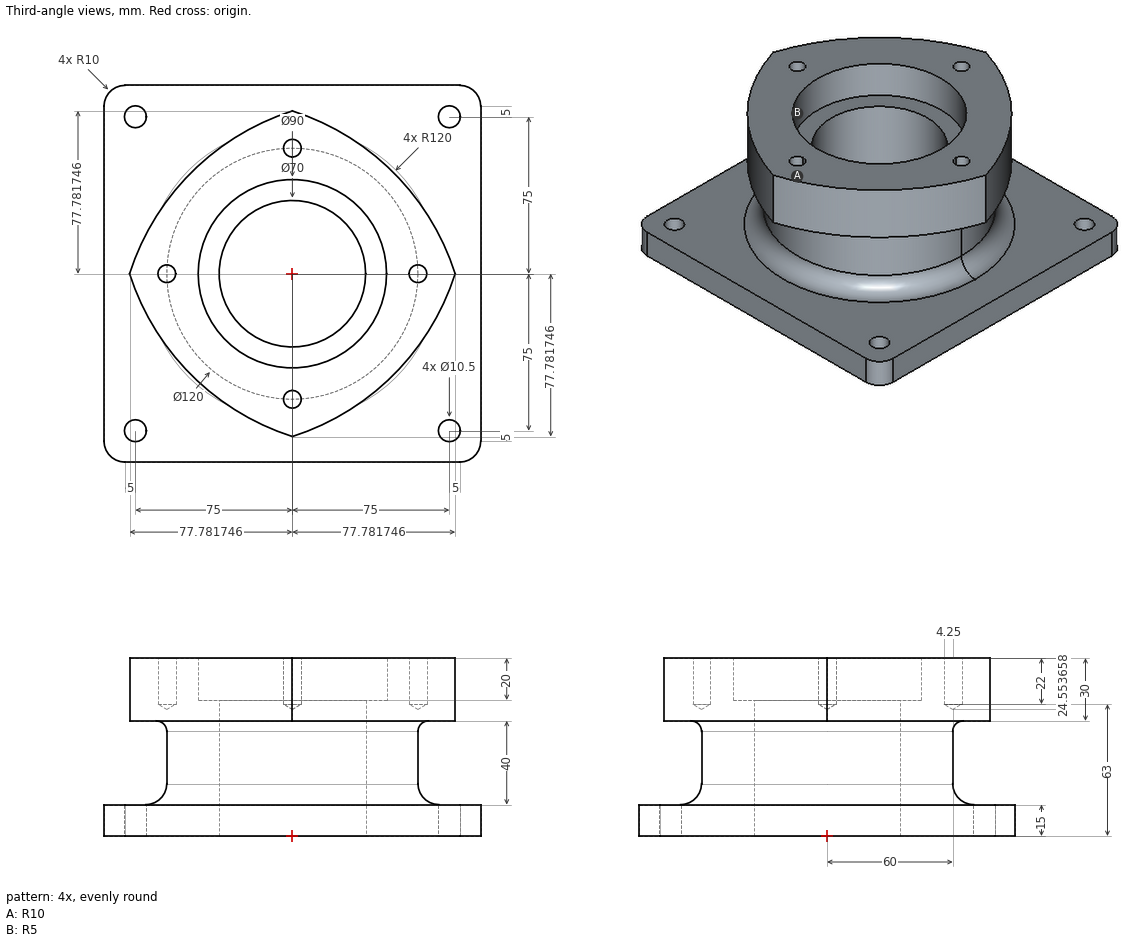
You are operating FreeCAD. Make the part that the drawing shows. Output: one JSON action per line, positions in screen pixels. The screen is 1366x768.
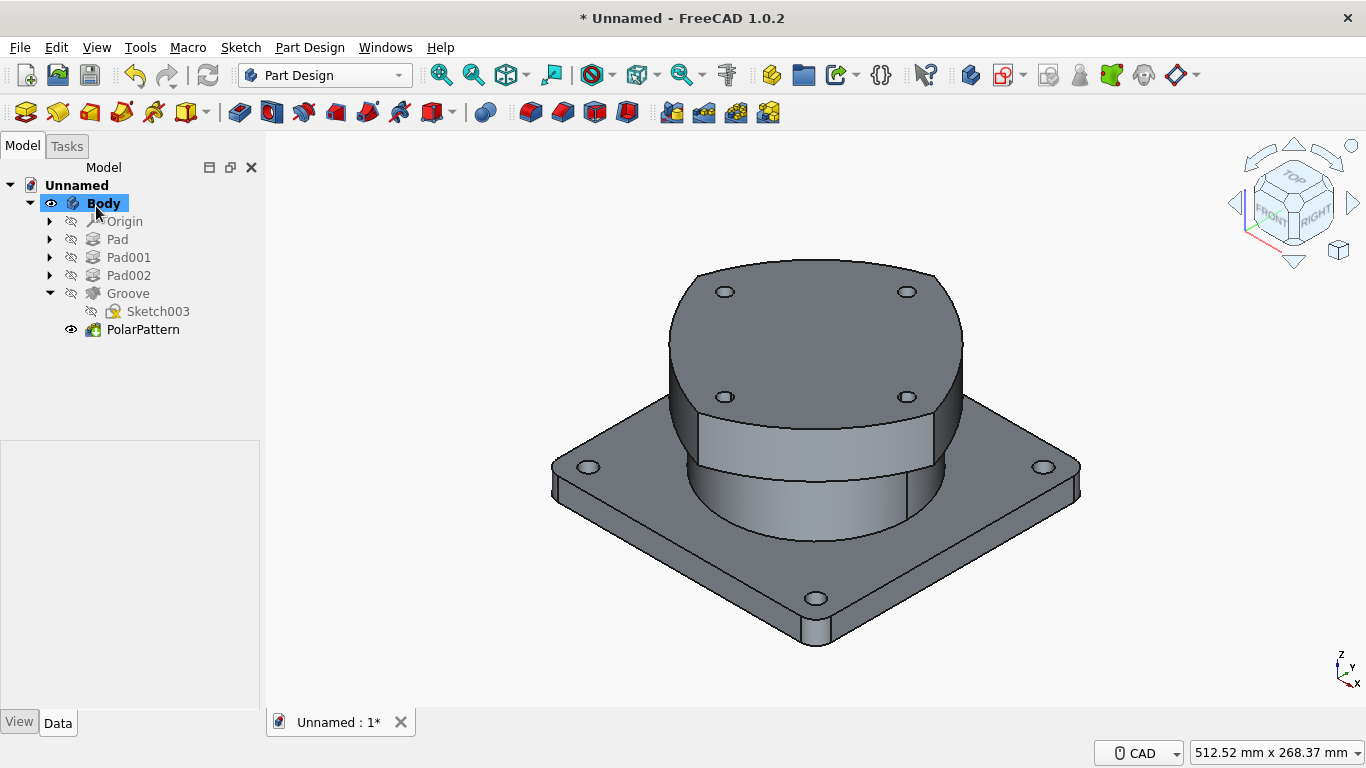
{"action": "key", "text": "2"}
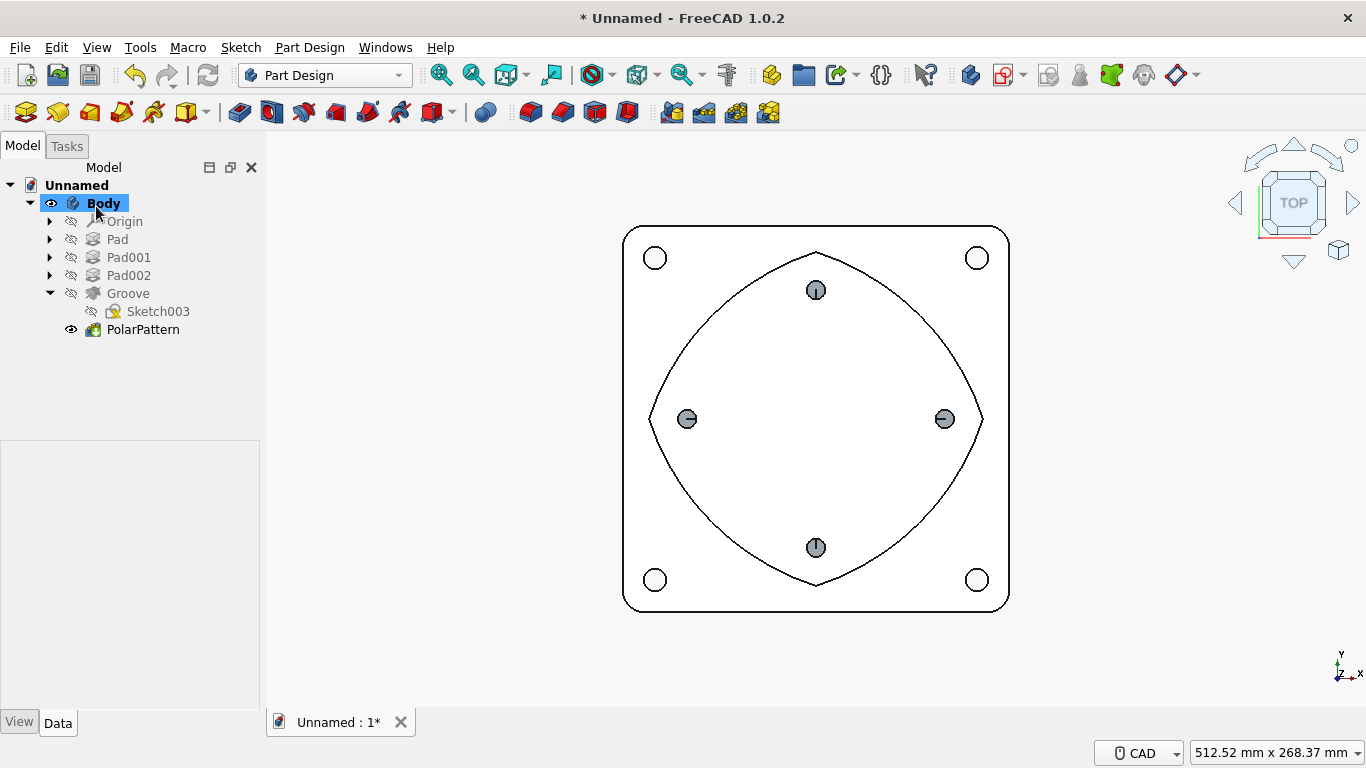
{"action": "key", "text": "1"}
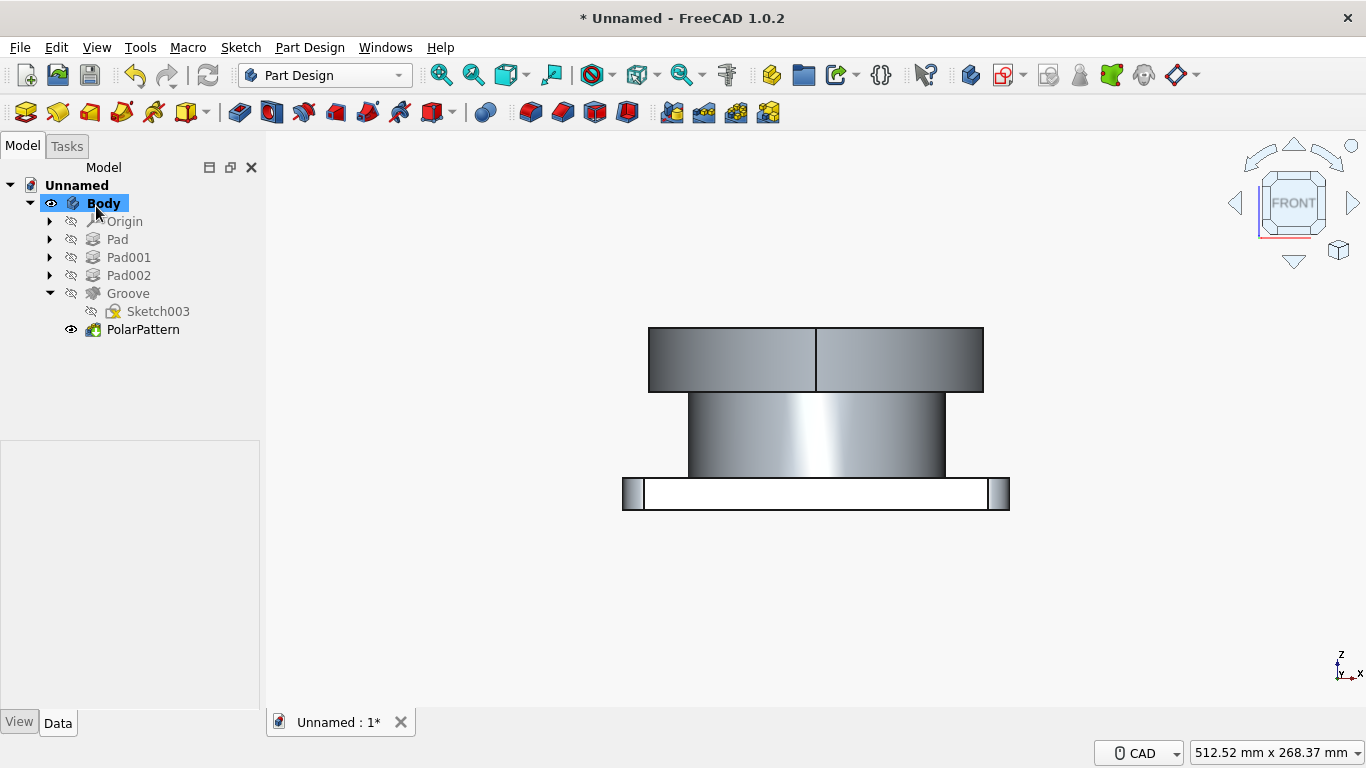
{"action": "left_click", "coordinate": [442, 76]}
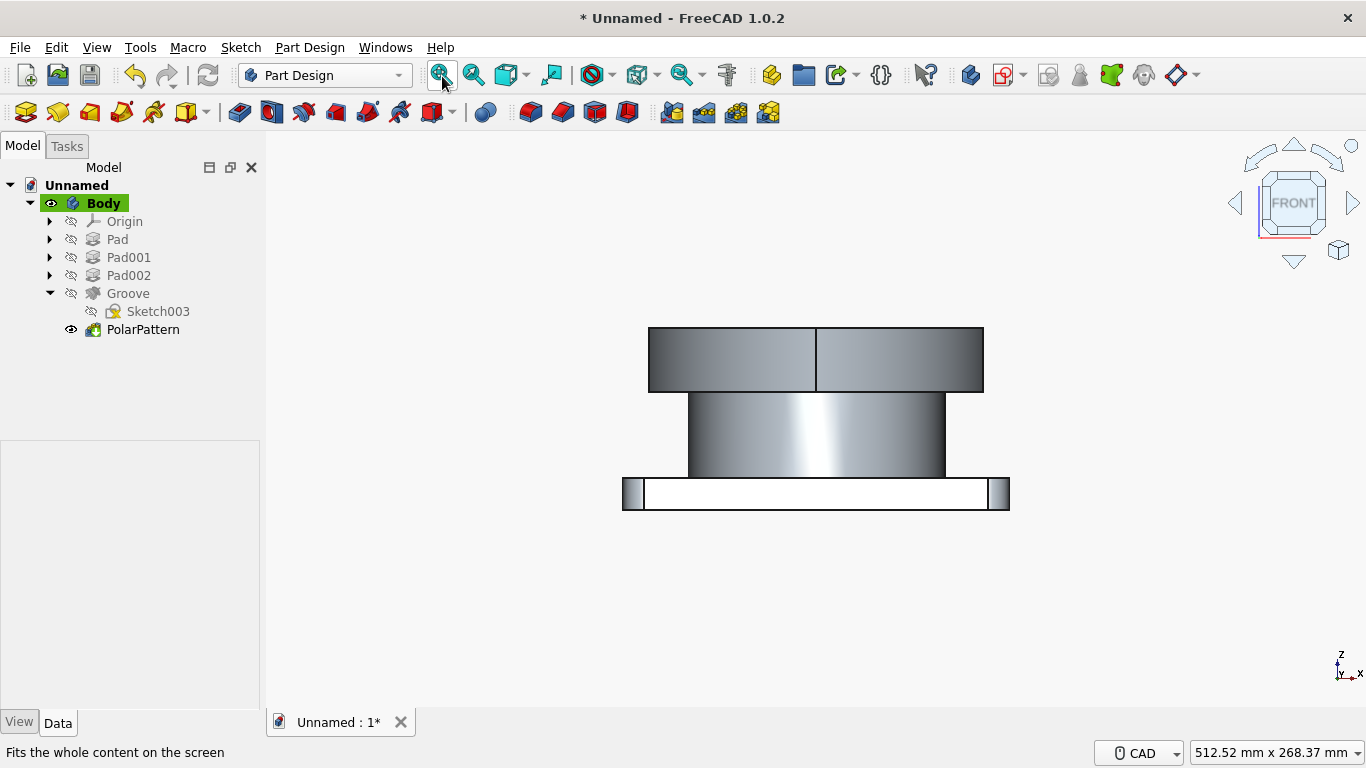
{"action": "key", "text": "3"}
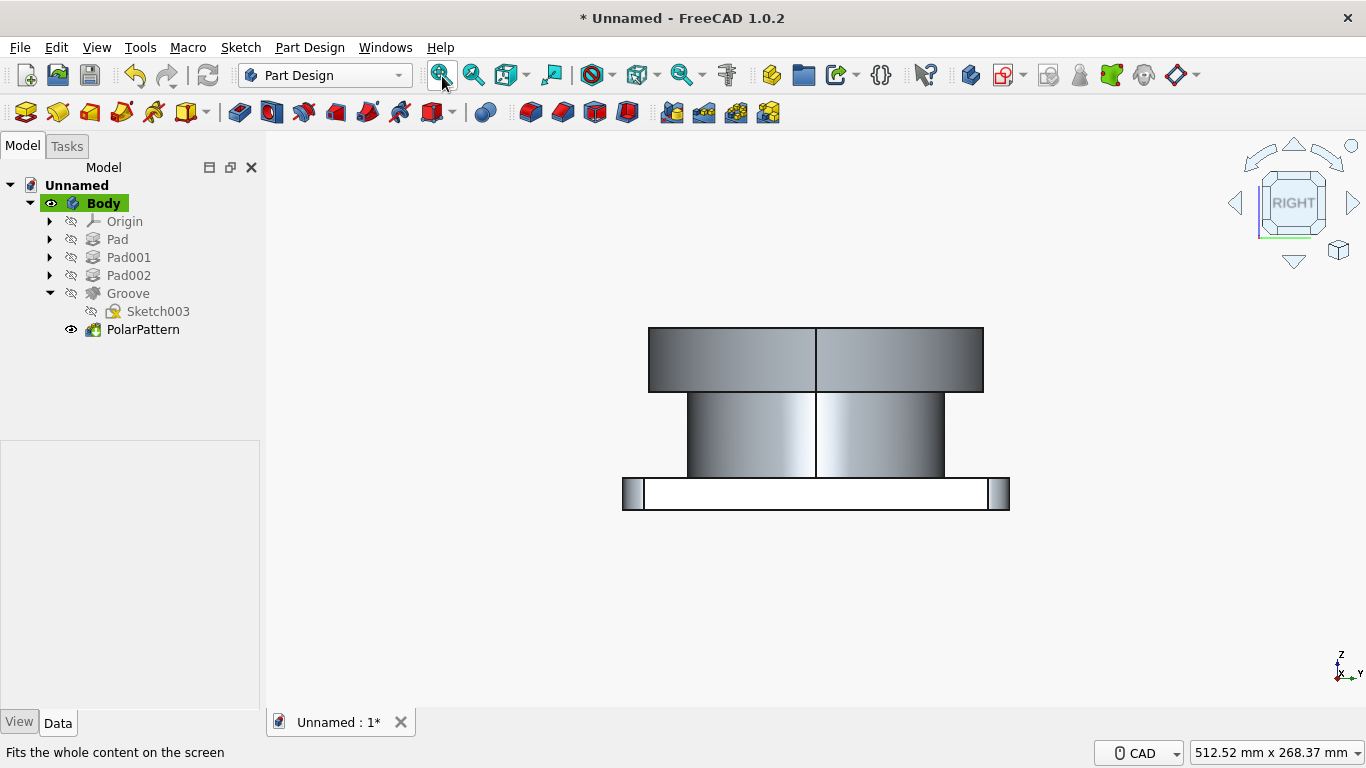
{"action": "left_click", "coordinate": [442, 76]}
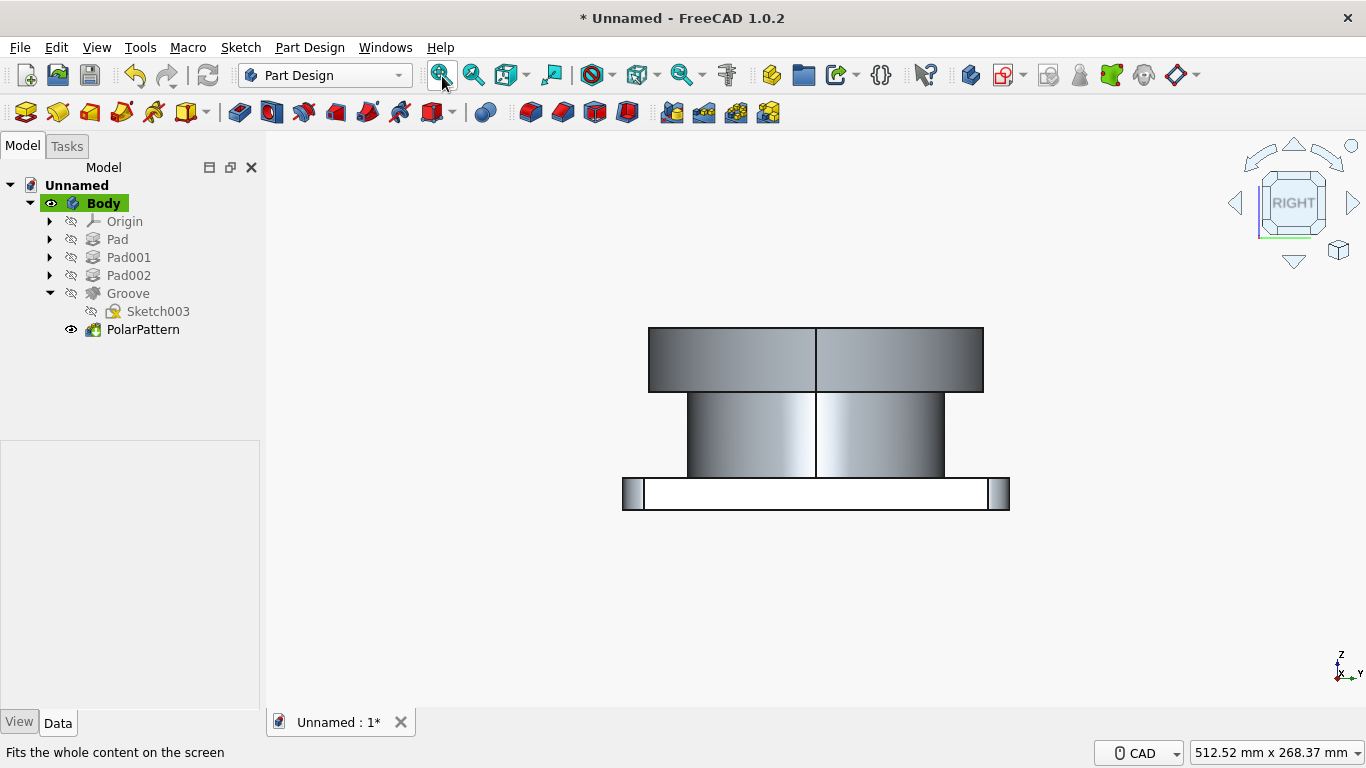
{"action": "key", "text": "5"}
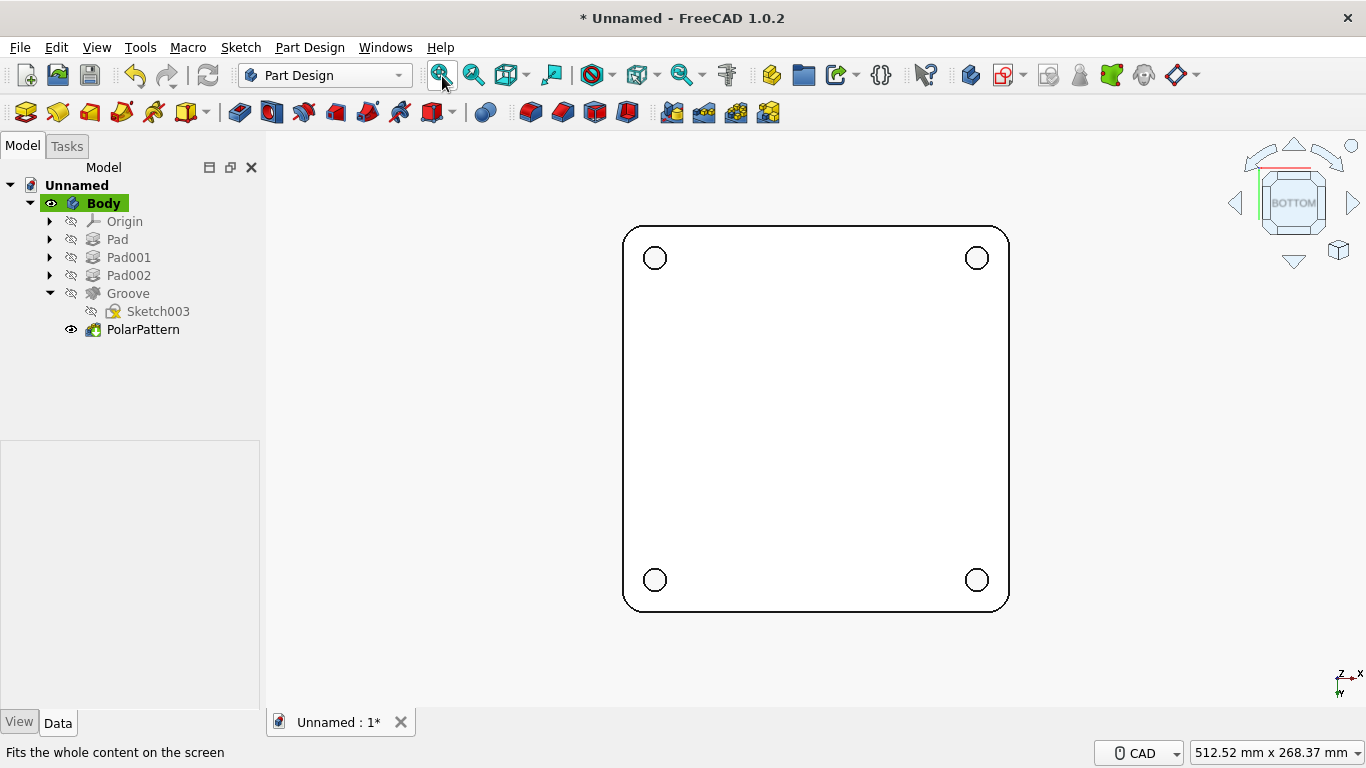
{"action": "key", "text": "4"}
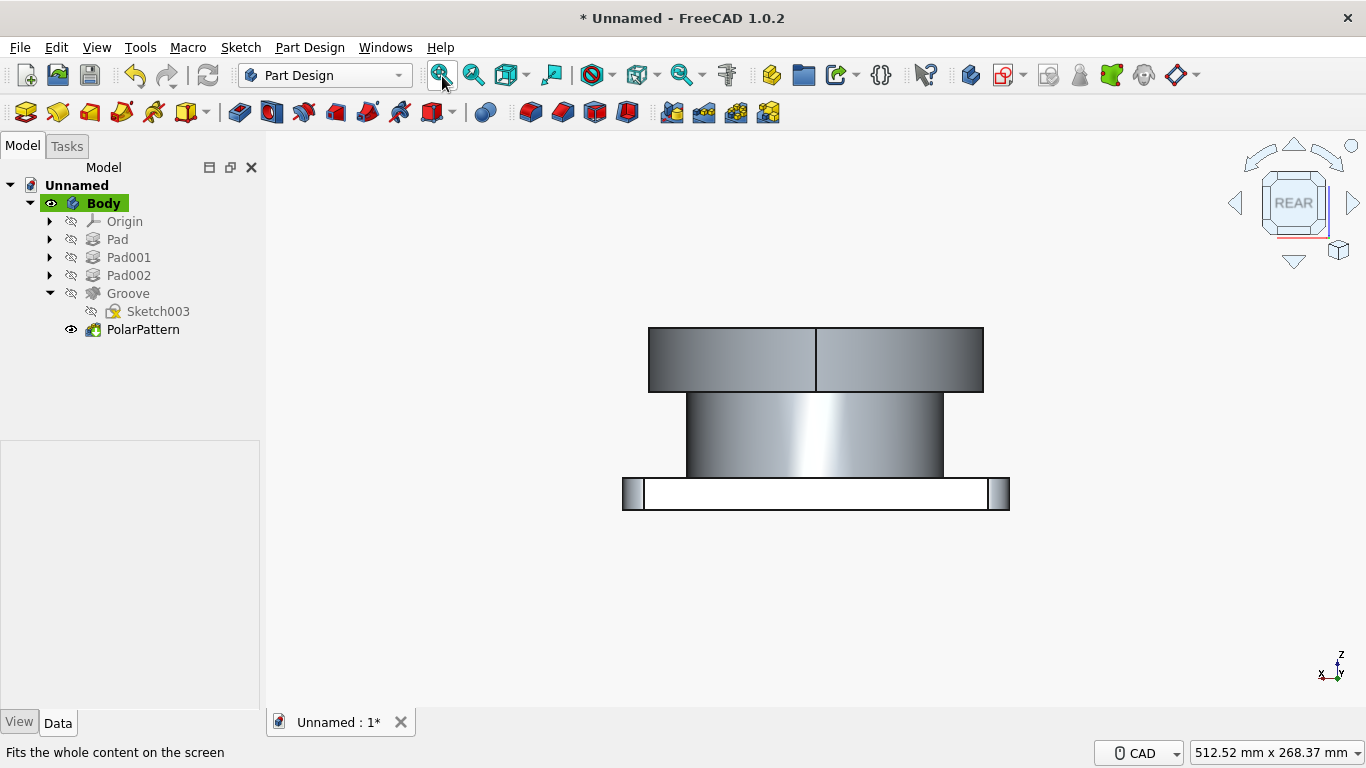
{"action": "left_click", "coordinate": [442, 76]}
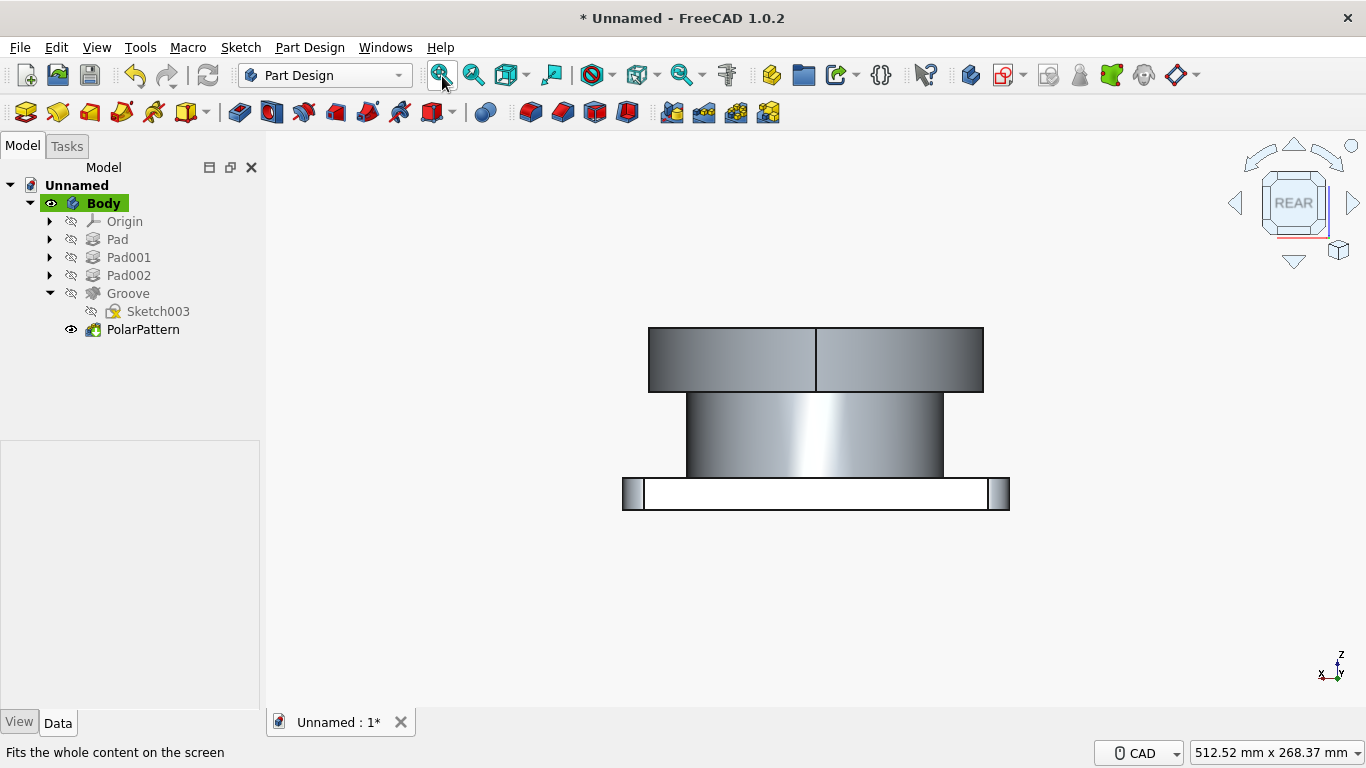
{"action": "key", "text": "6"}